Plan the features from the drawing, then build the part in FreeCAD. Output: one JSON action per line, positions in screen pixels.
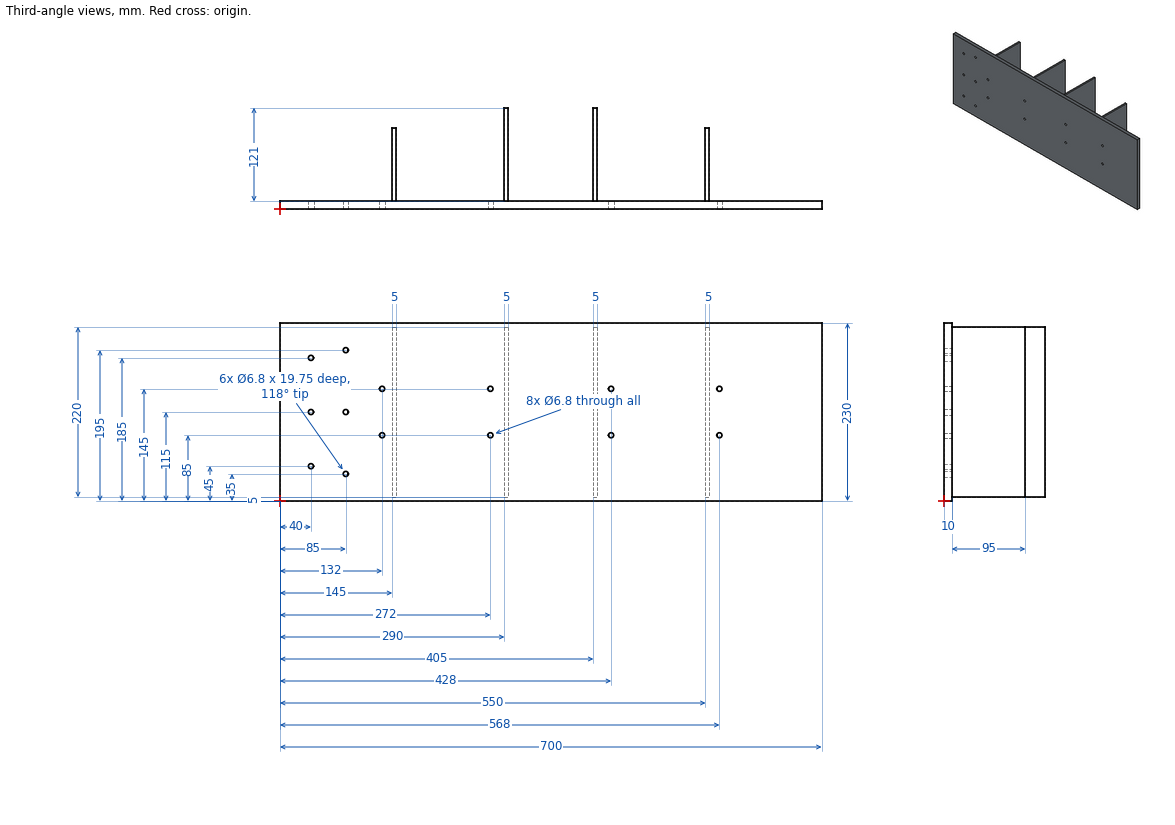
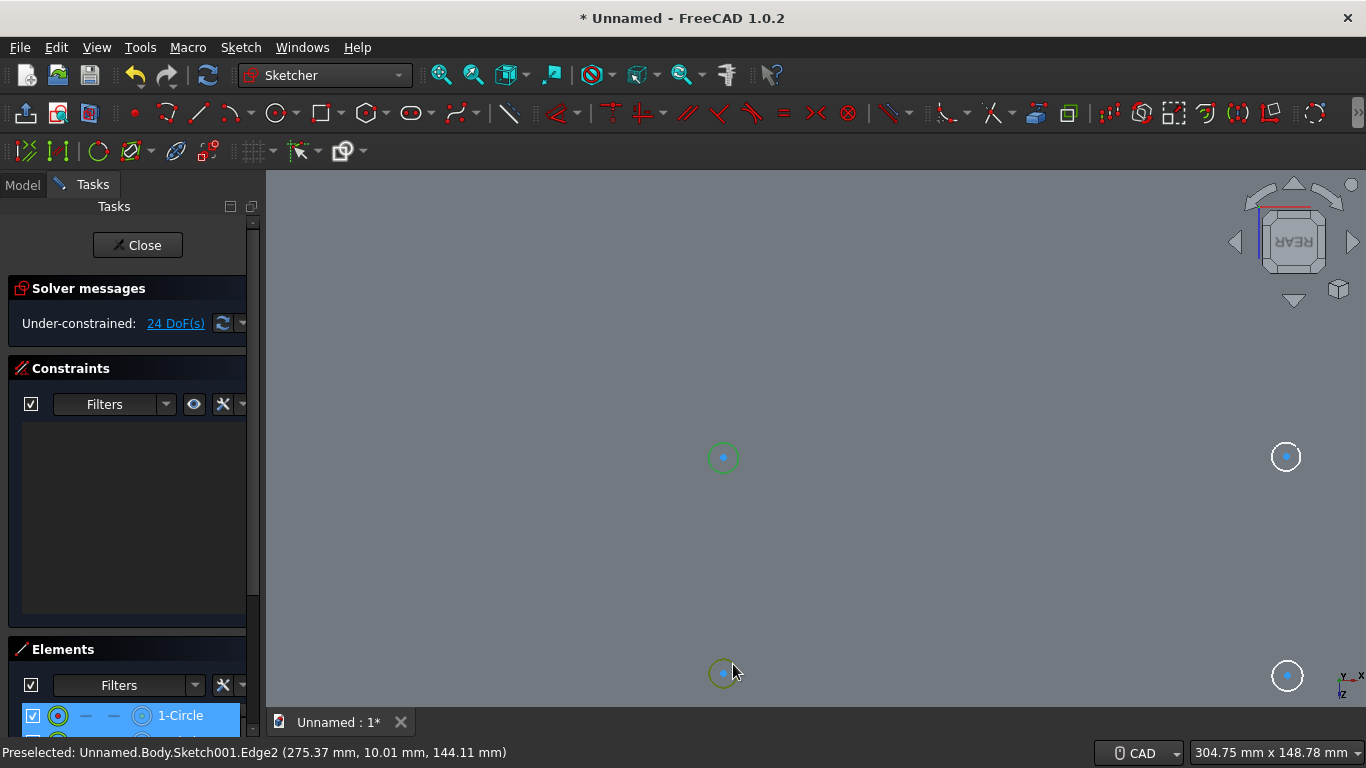
{"action": "scroll", "coordinate": [736, 448], "scroll_direction": "down", "scroll_amount": 6}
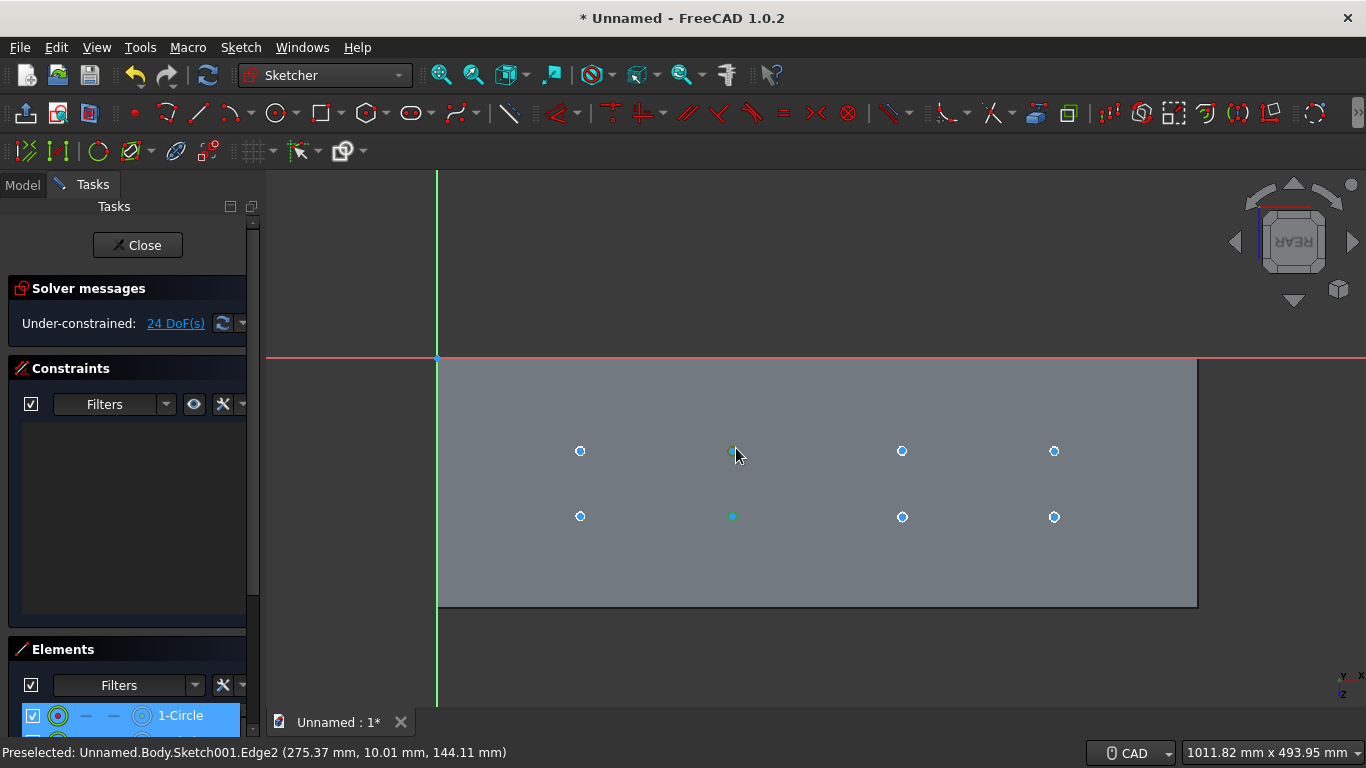
{"action": "scroll", "coordinate": [583, 513], "scroll_direction": "up", "scroll_amount": 7}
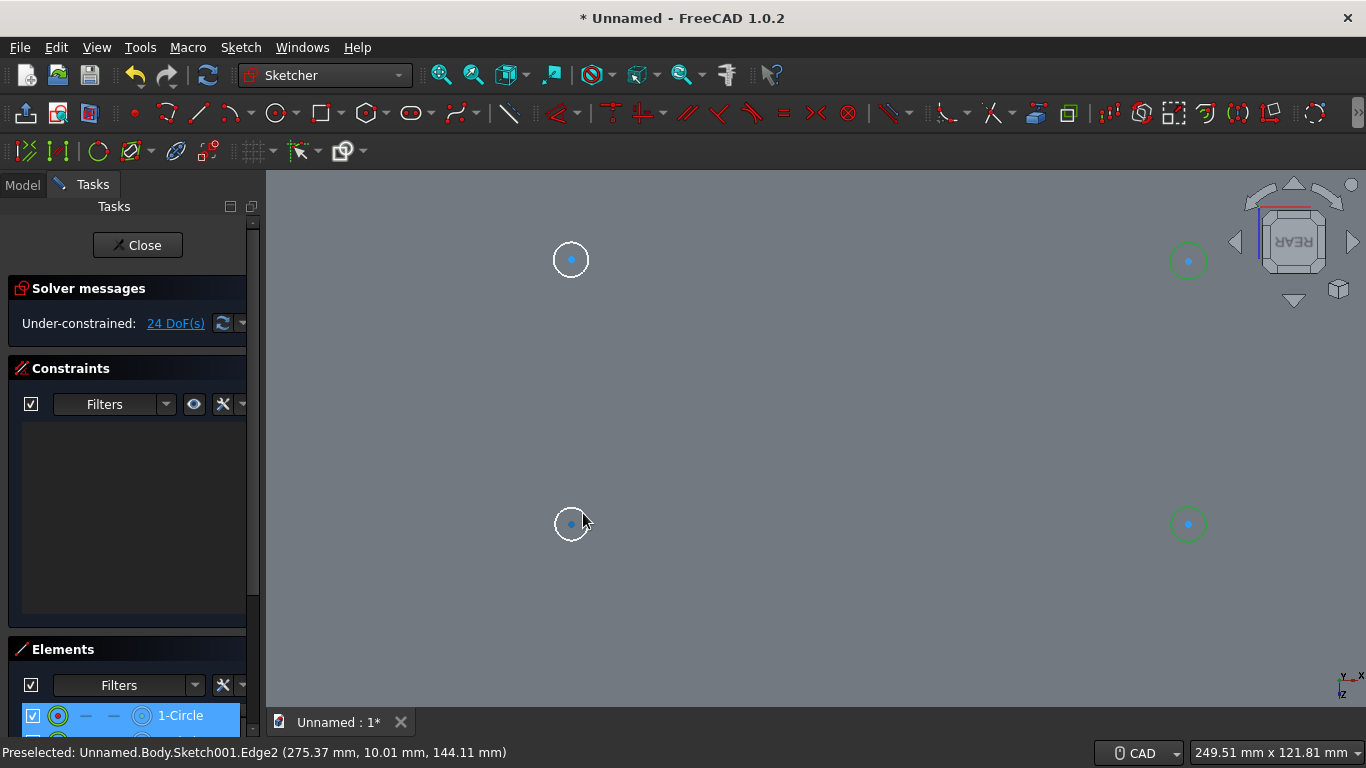
{"action": "left_click", "coordinate": [583, 513]}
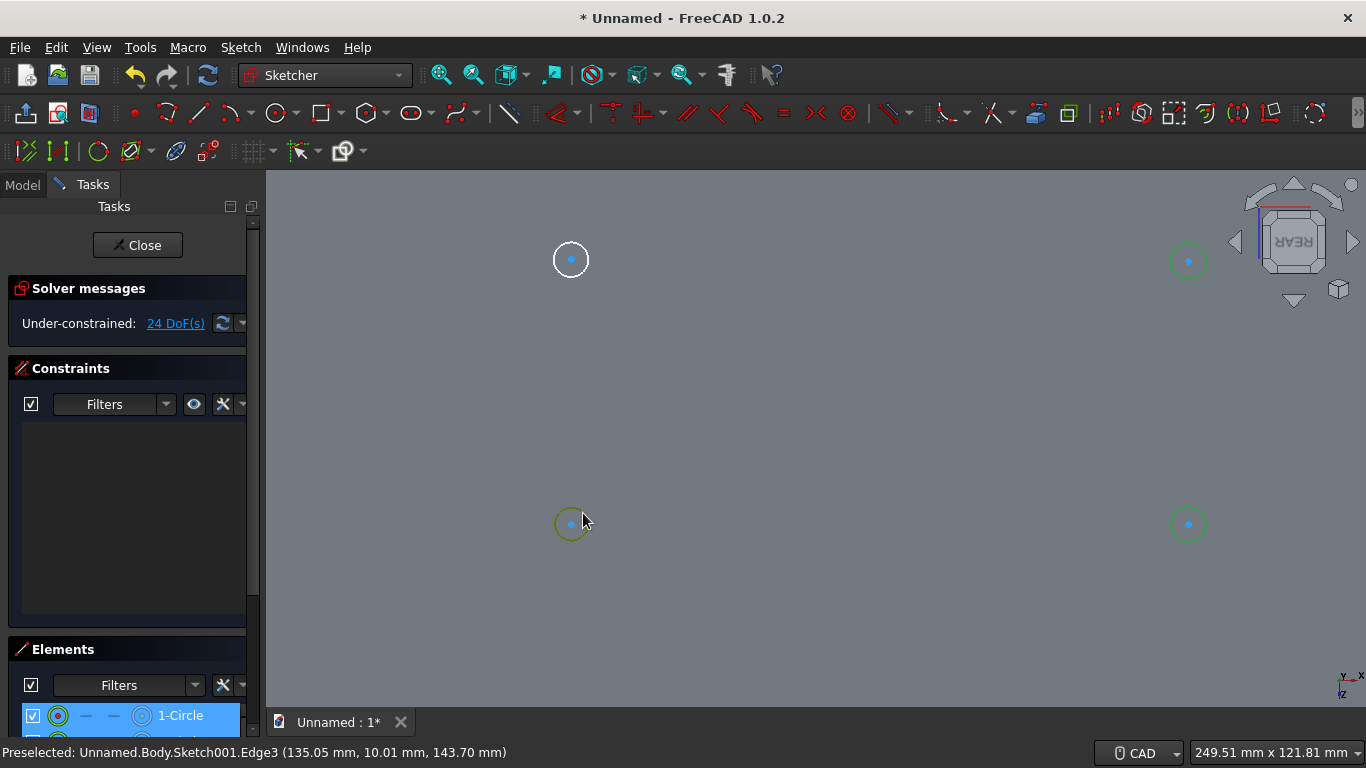
{"action": "left_click", "coordinate": [583, 247]}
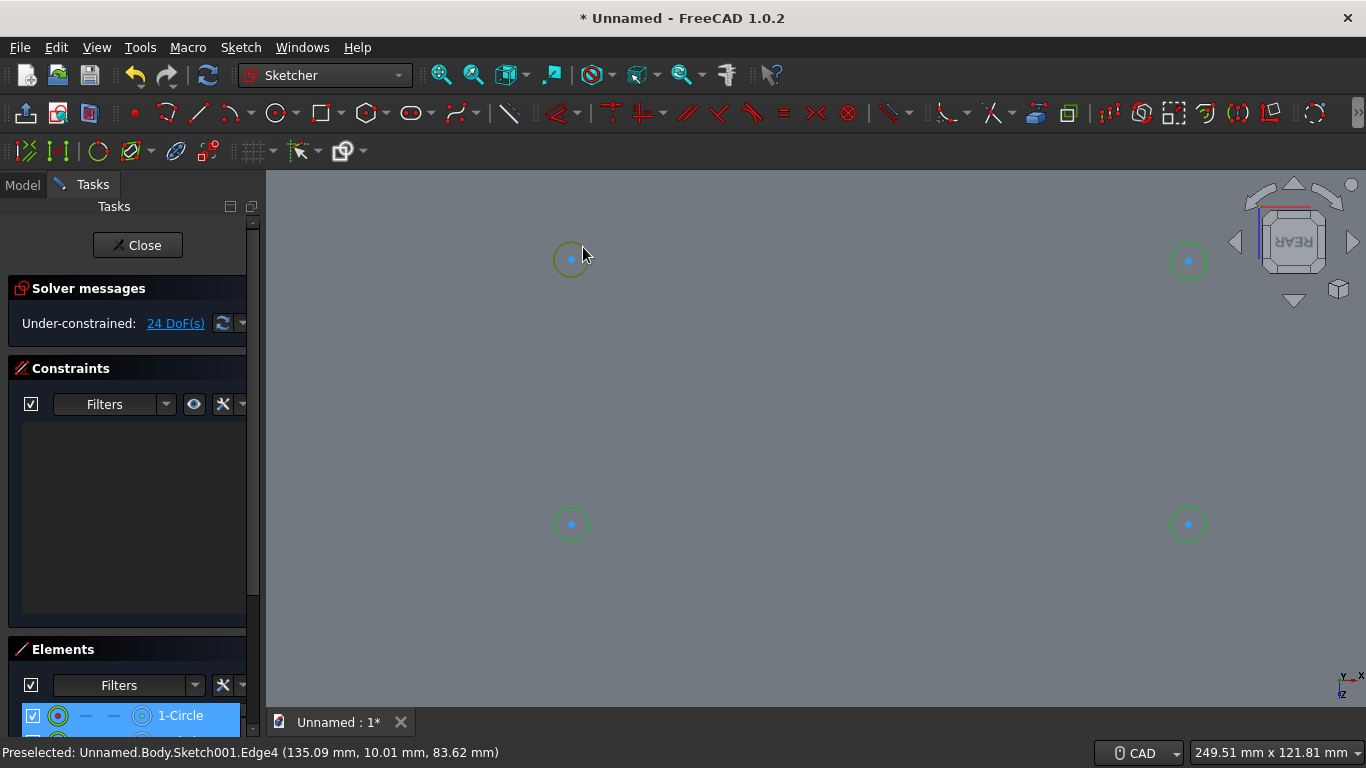
{"action": "scroll", "coordinate": [583, 513], "scroll_direction": "down", "scroll_amount": 7}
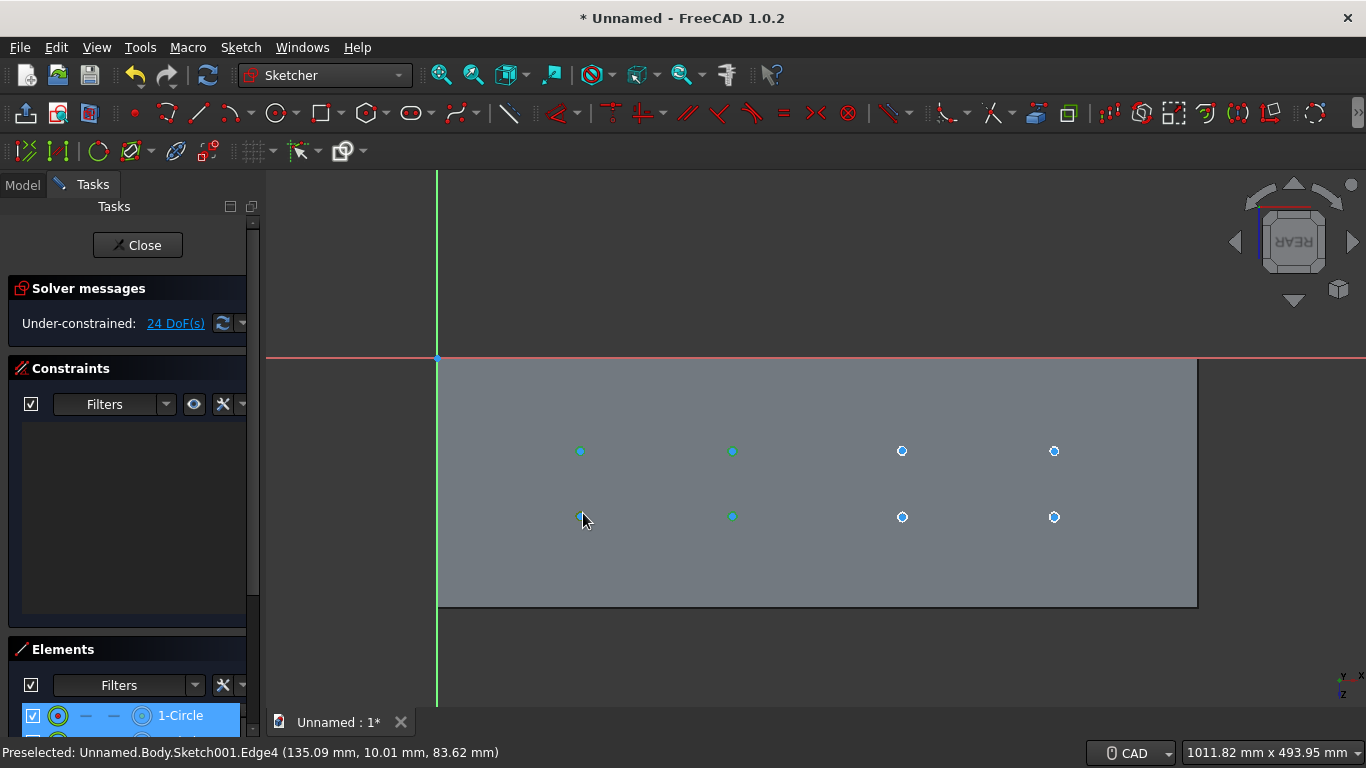
{"action": "scroll", "coordinate": [1057, 448], "scroll_direction": "up", "scroll_amount": 7}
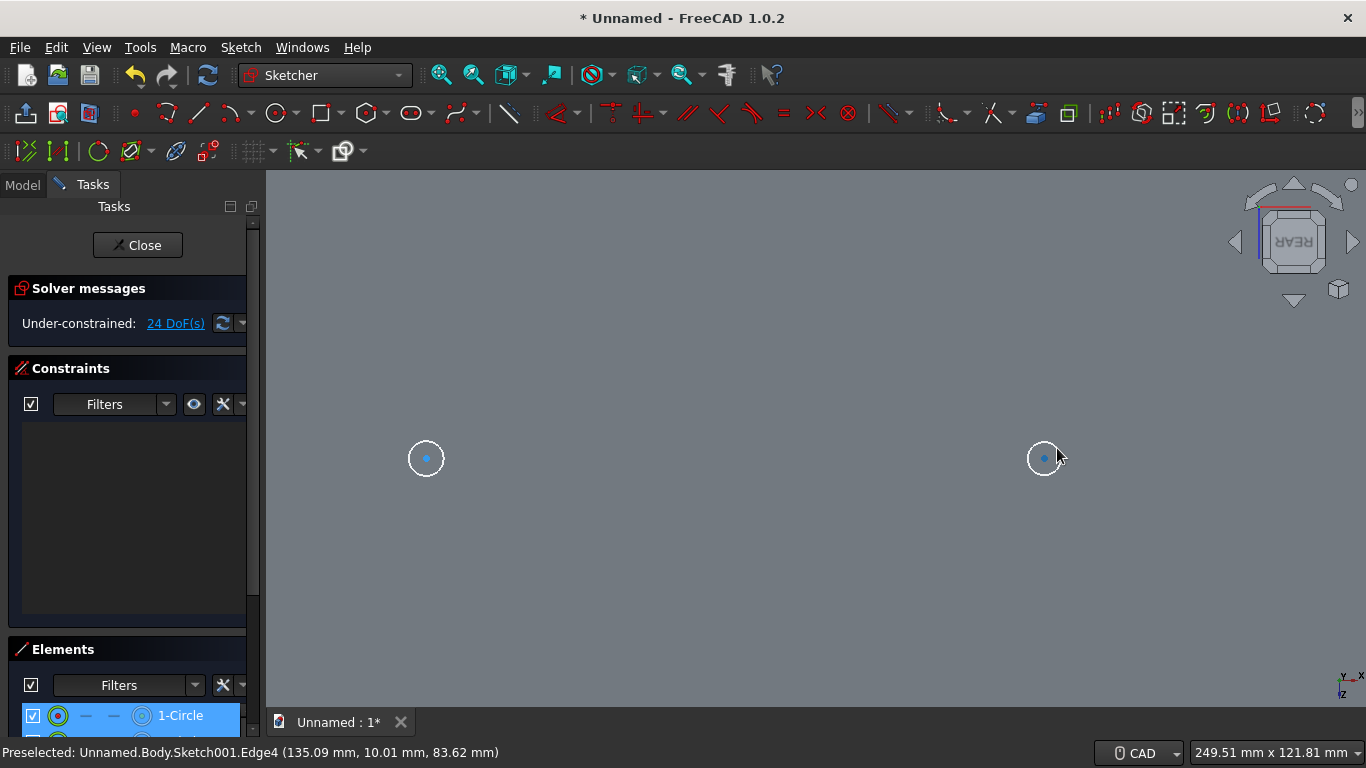
{"action": "left_click", "coordinate": [1056, 447]}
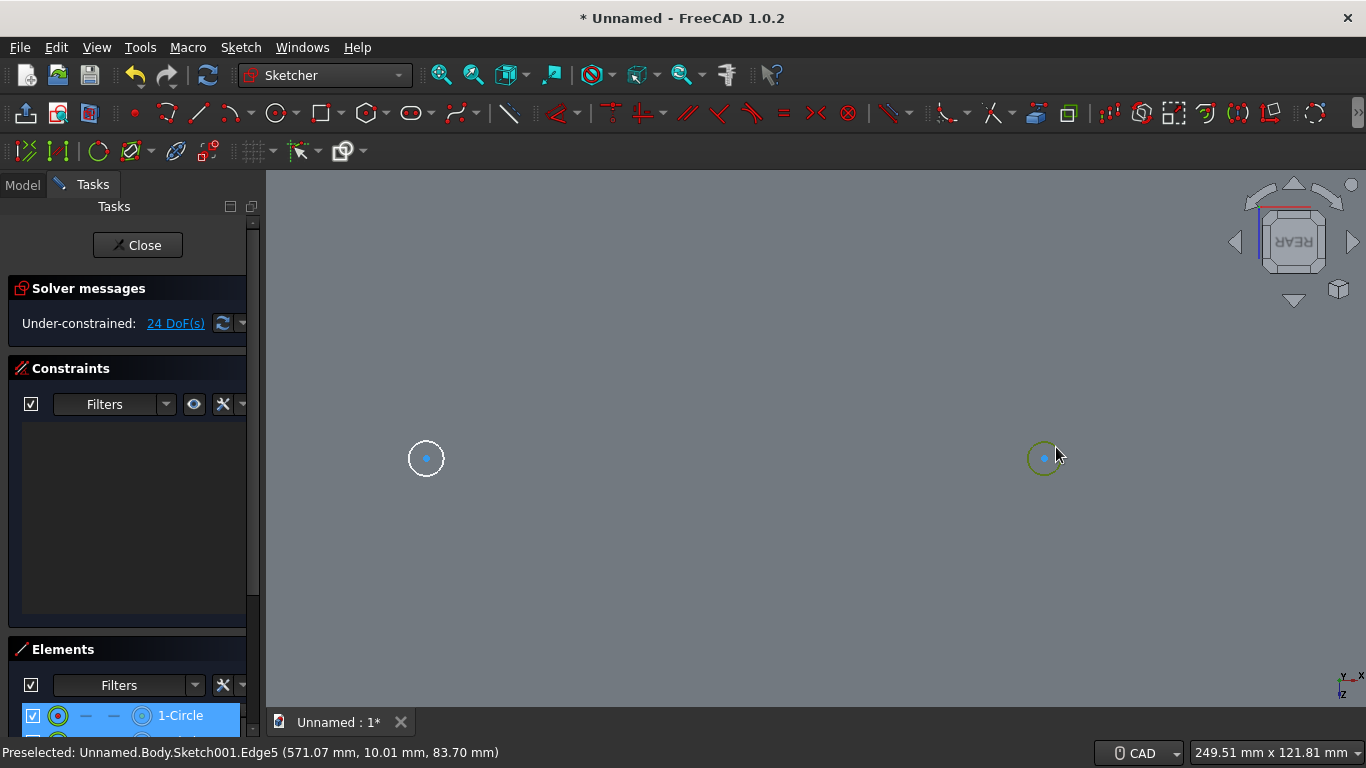
{"action": "scroll", "coordinate": [1057, 448], "scroll_direction": "down", "scroll_amount": 7}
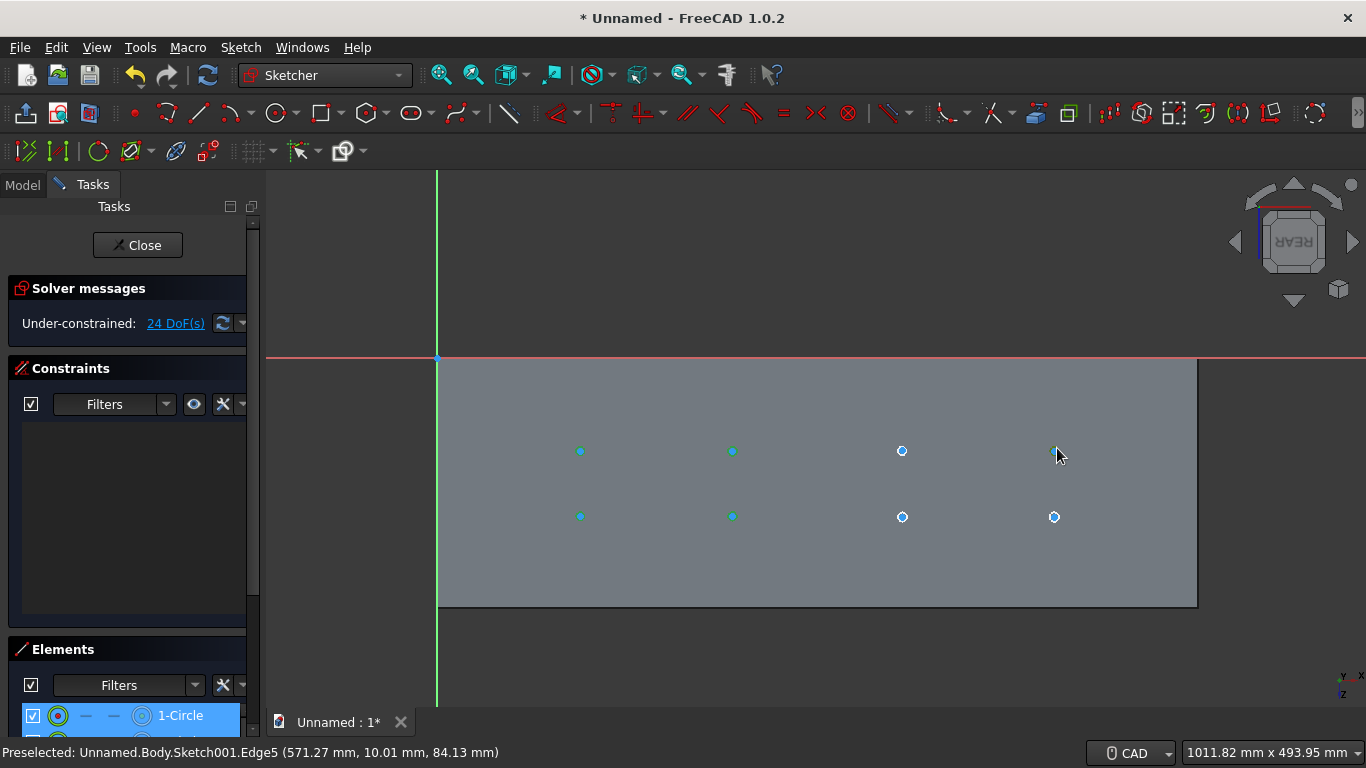
{"action": "scroll", "coordinate": [1058, 514], "scroll_direction": "up", "scroll_amount": 6}